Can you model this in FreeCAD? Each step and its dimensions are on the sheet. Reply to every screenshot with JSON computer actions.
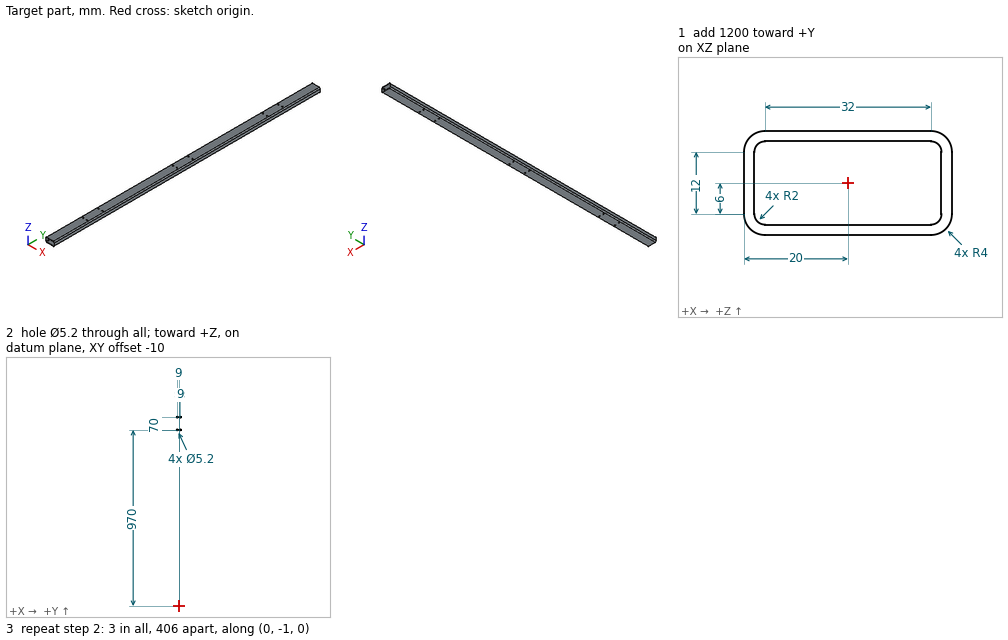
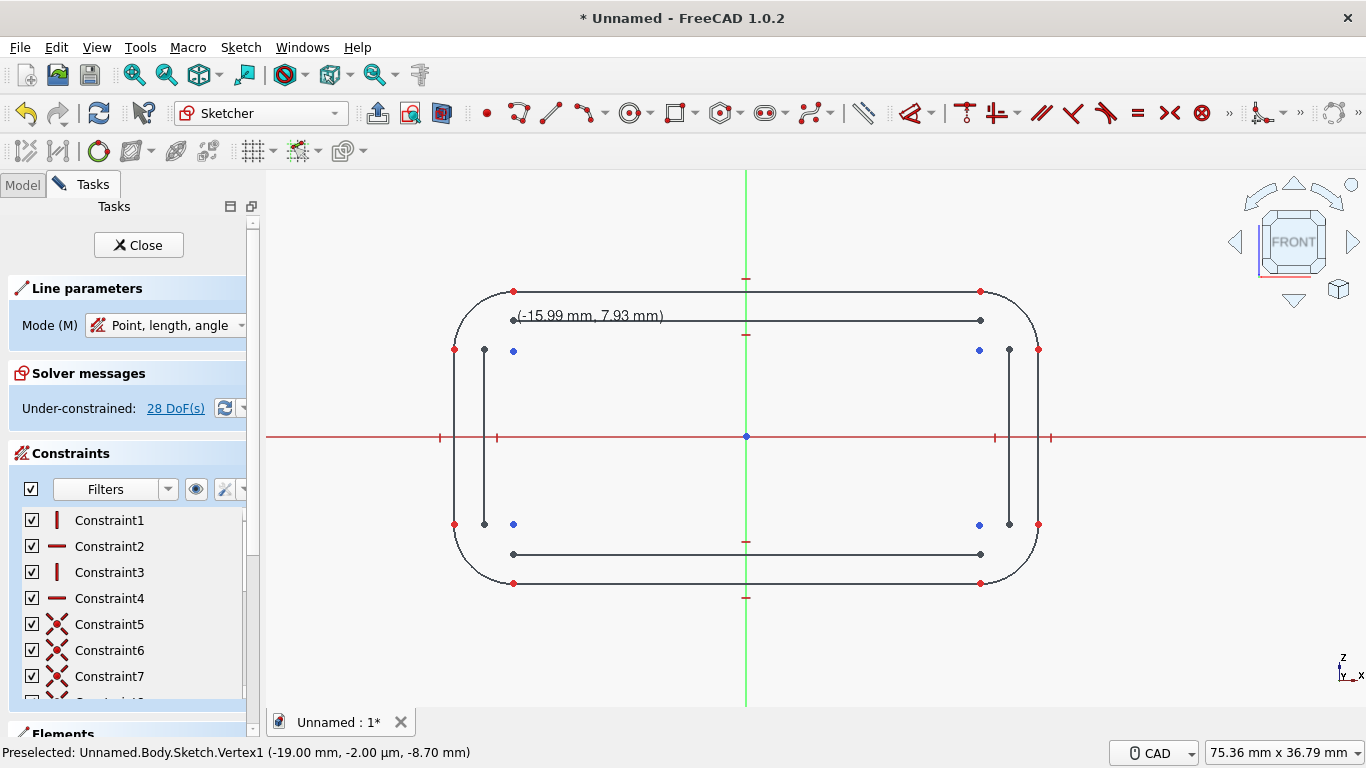
{"action": "left_click", "coordinate": [584, 114]}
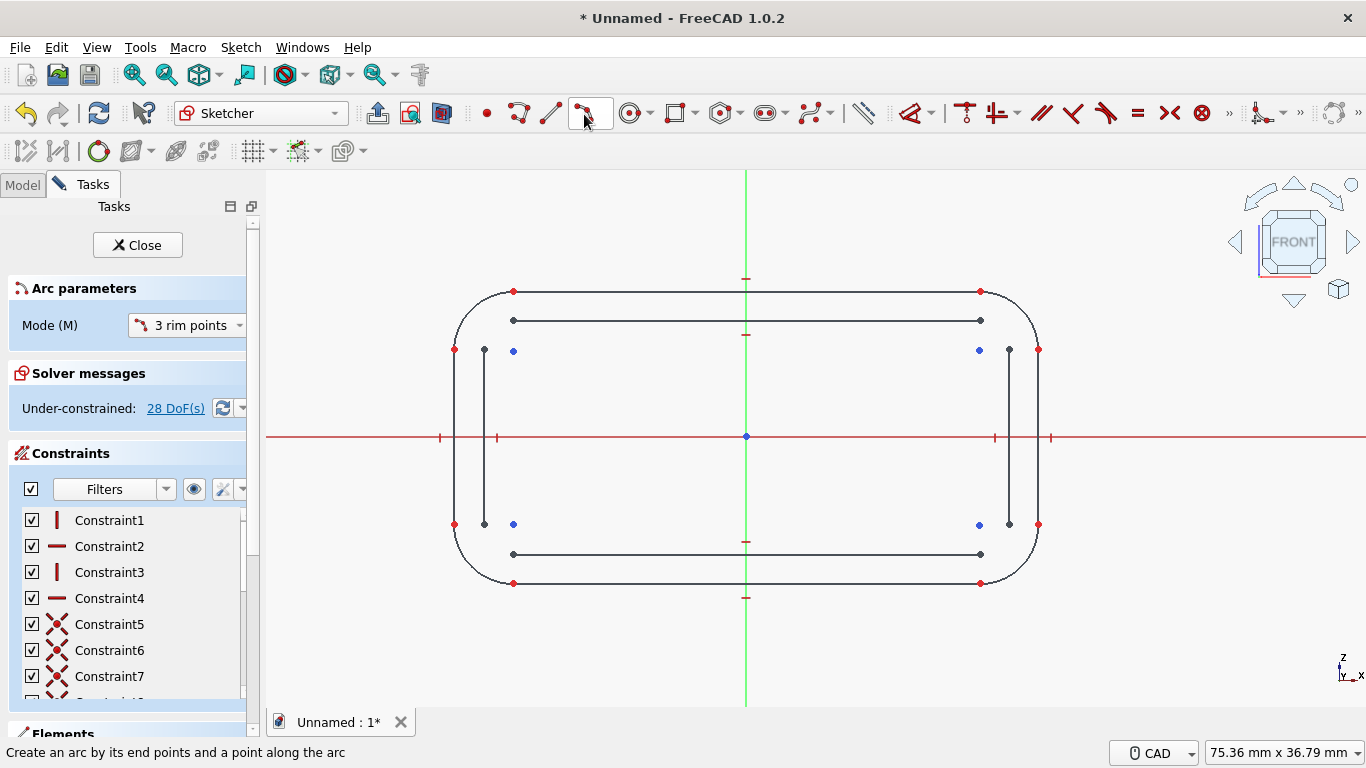
{"action": "left_click", "coordinate": [484, 525]}
{"action": "left_click", "coordinate": [513, 555]}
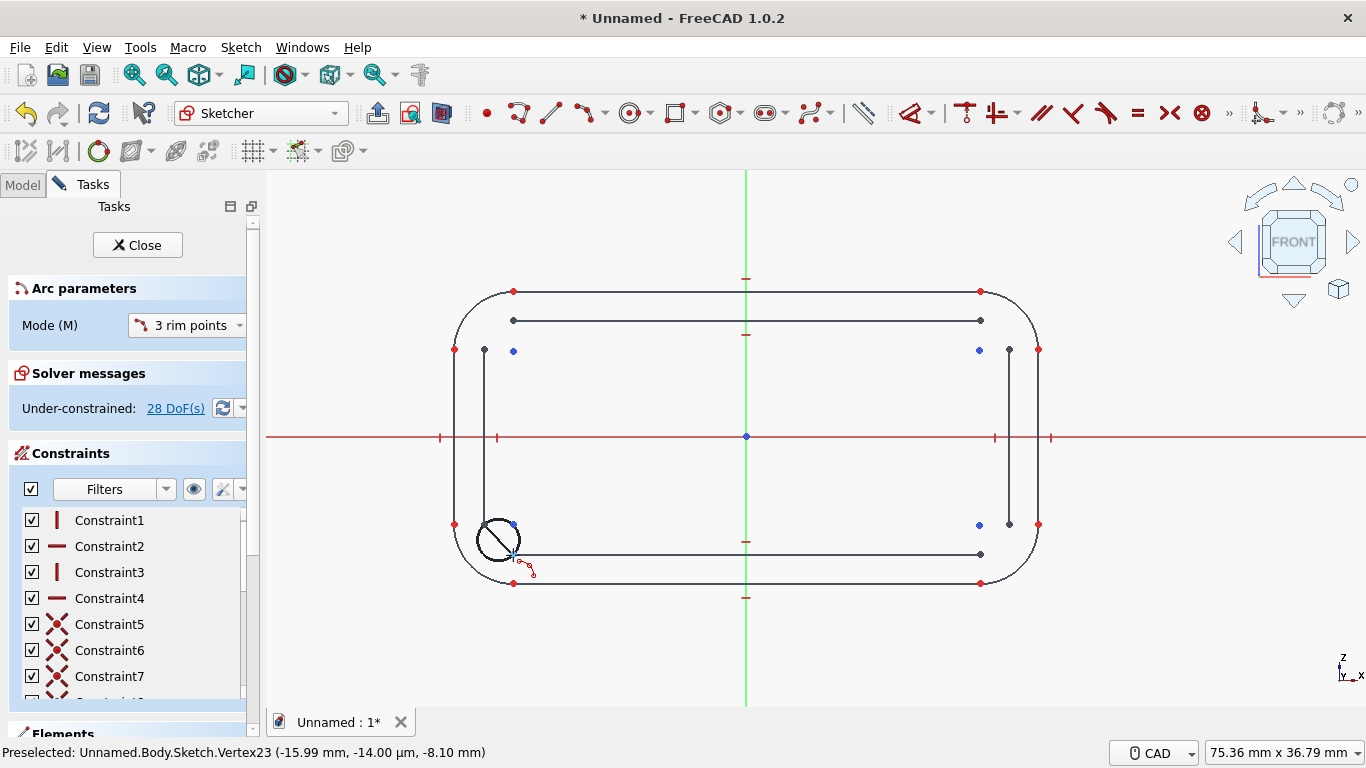
{"action": "scroll", "coordinate": [492, 545], "scroll_direction": "up", "scroll_amount": 4}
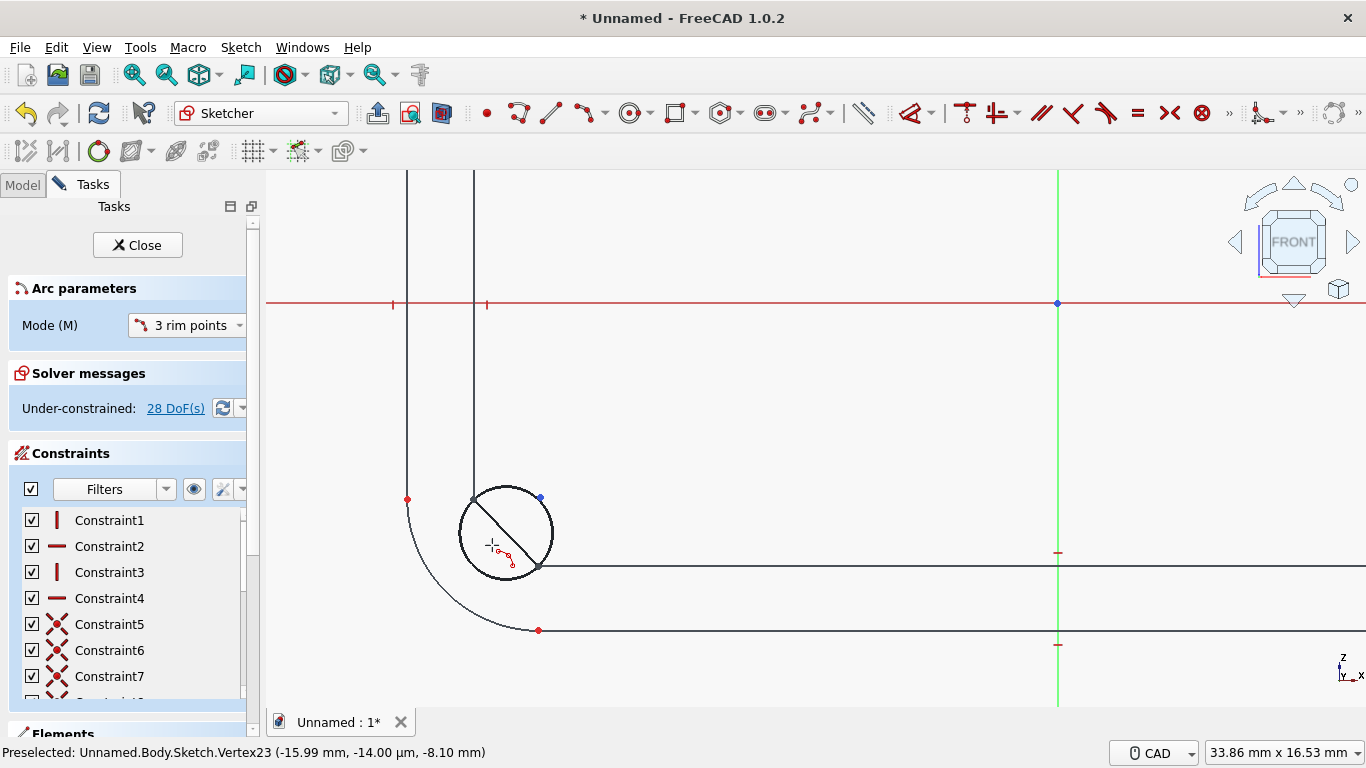
{"action": "left_click", "coordinate": [492, 544]}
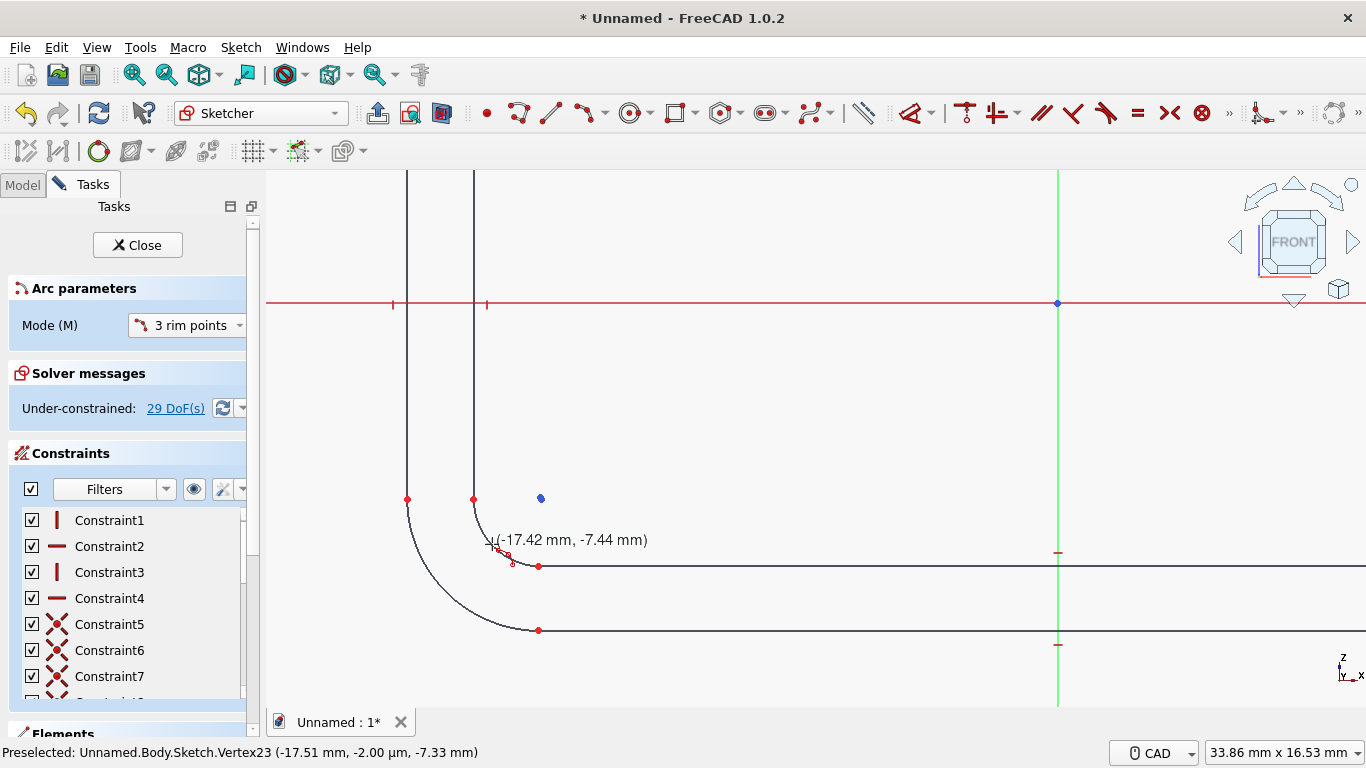
{"action": "scroll", "coordinate": [494, 549], "scroll_direction": "down", "scroll_amount": 4}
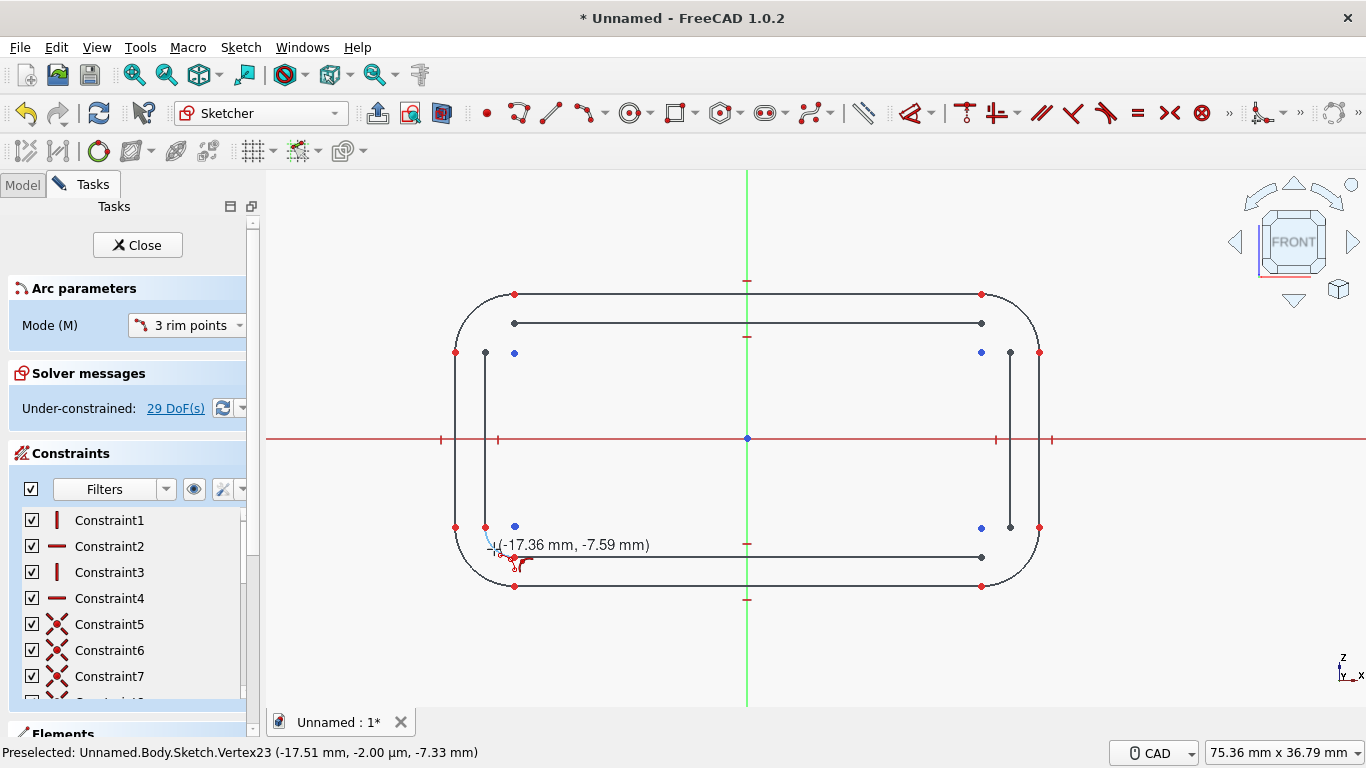
{"action": "left_click", "coordinate": [981, 557]}
{"action": "left_click", "coordinate": [1010, 527]}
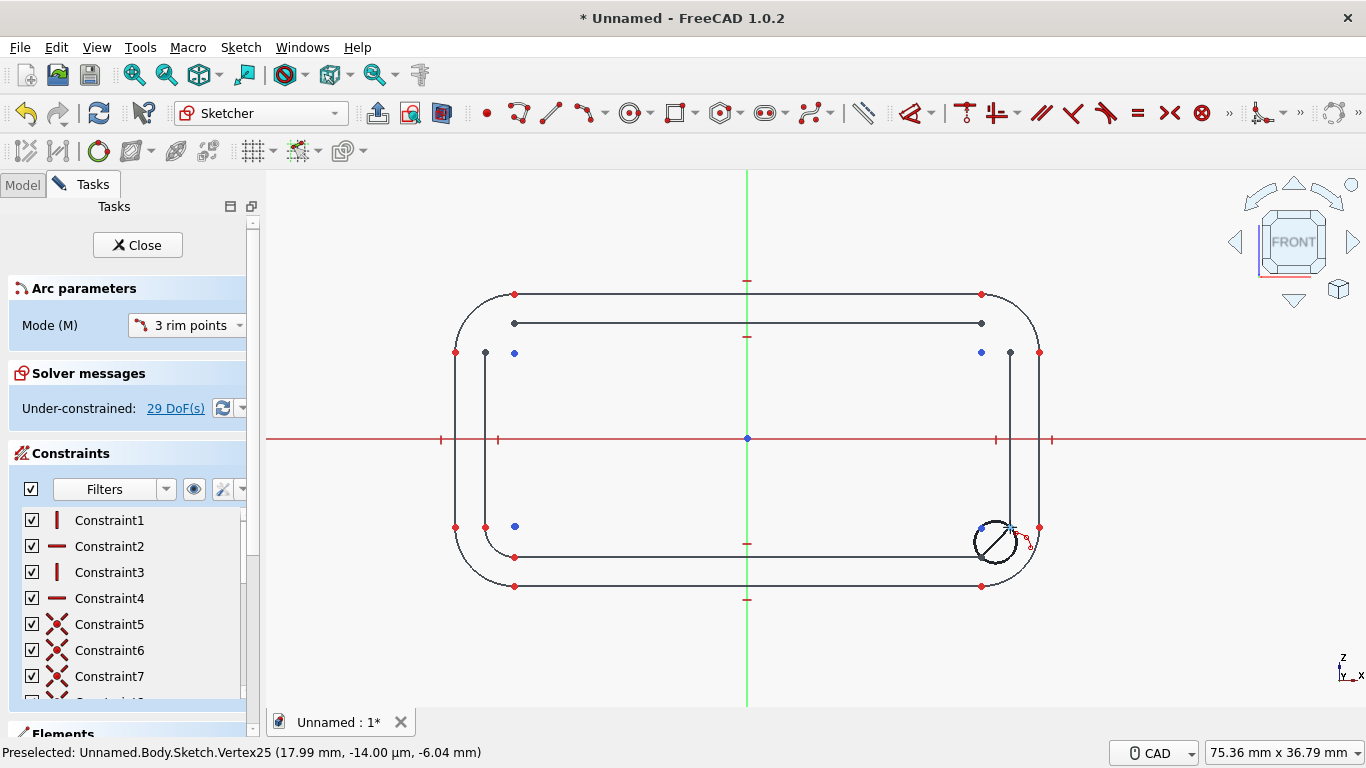
{"action": "scroll", "coordinate": [1002, 547], "scroll_direction": "up", "scroll_amount": 4}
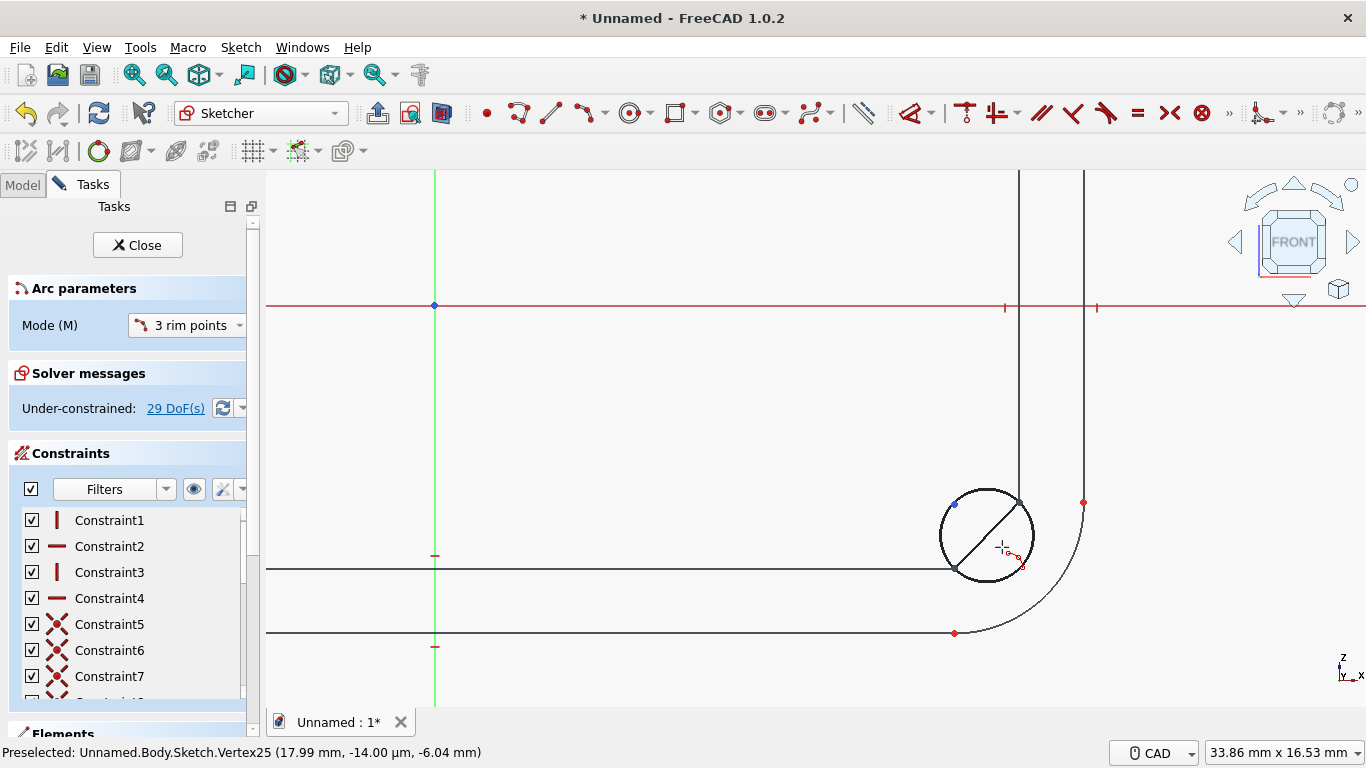
{"action": "left_click", "coordinate": [1000, 547]}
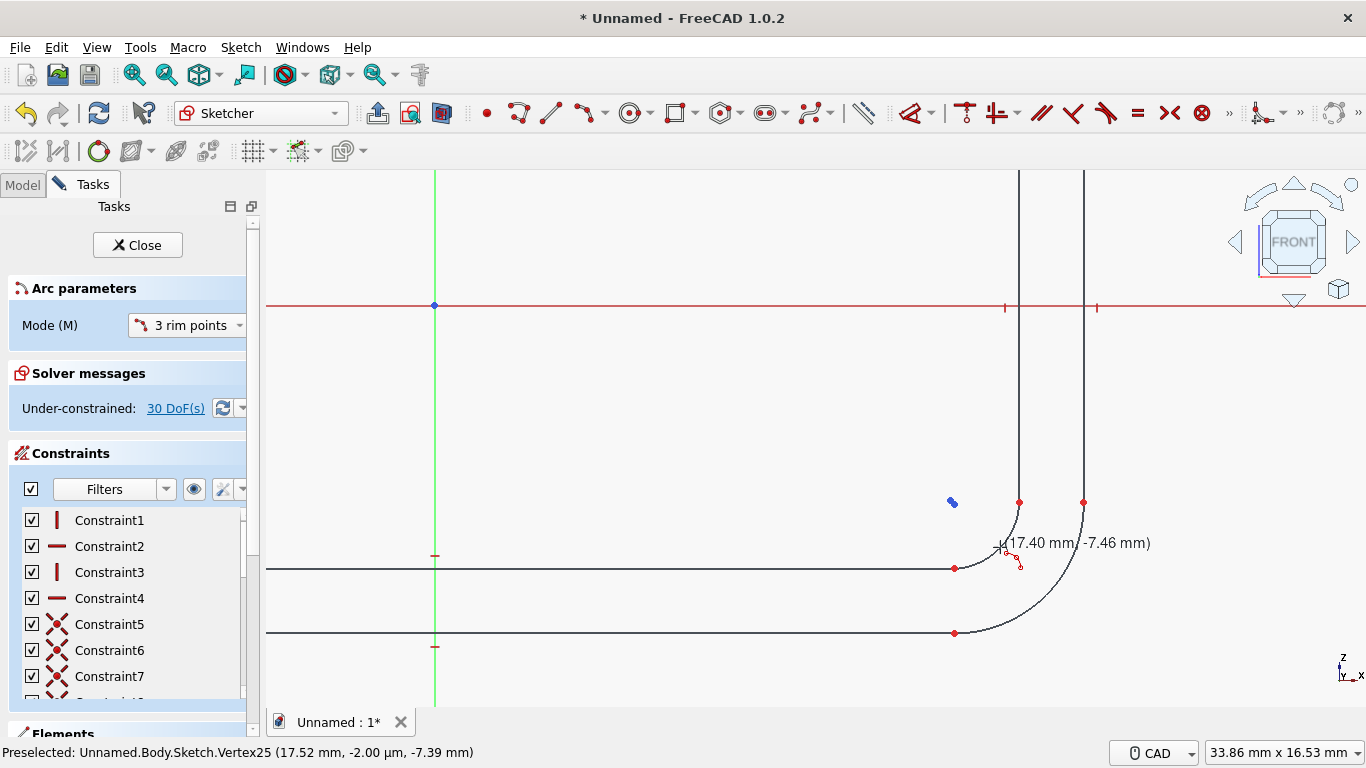
{"action": "scroll", "coordinate": [1003, 547], "scroll_direction": "down", "scroll_amount": 4}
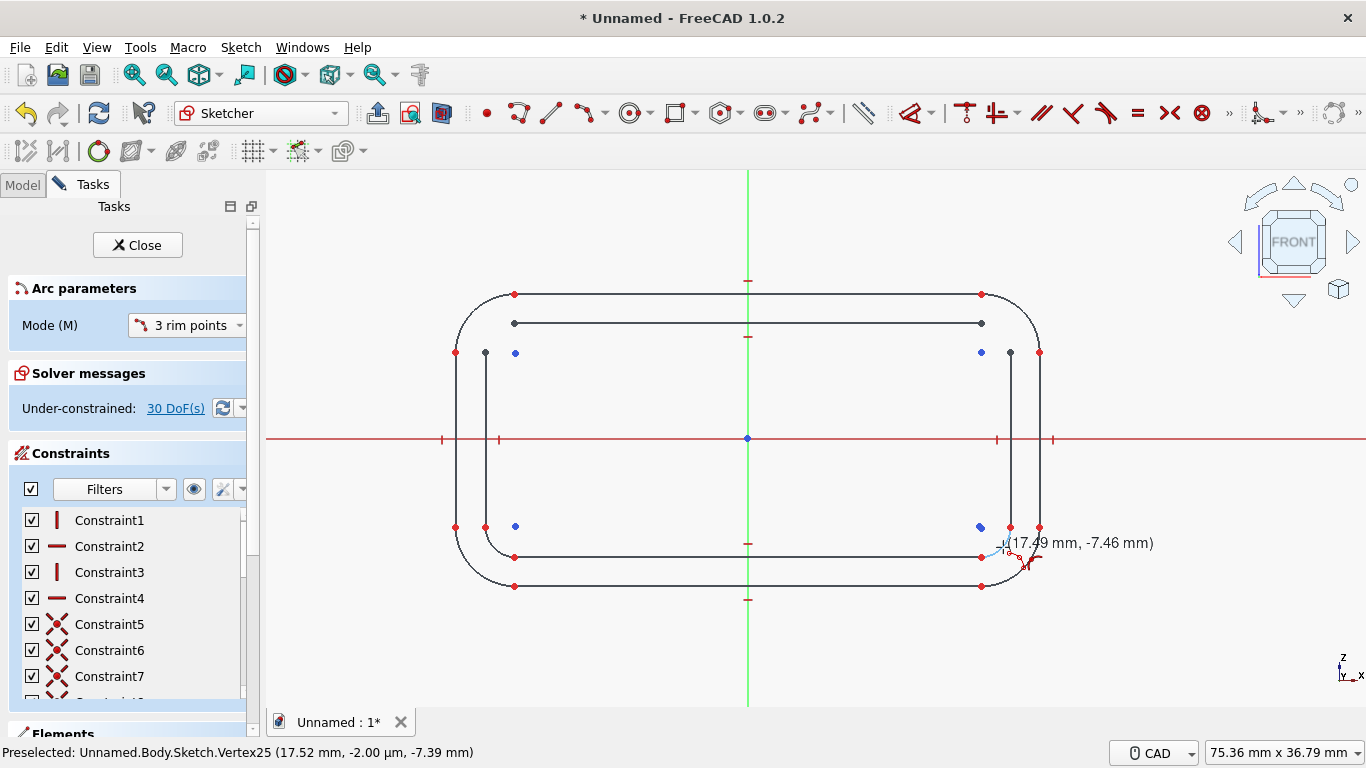
{"action": "left_click", "coordinate": [1011, 352]}
{"action": "left_click", "coordinate": [982, 323]}